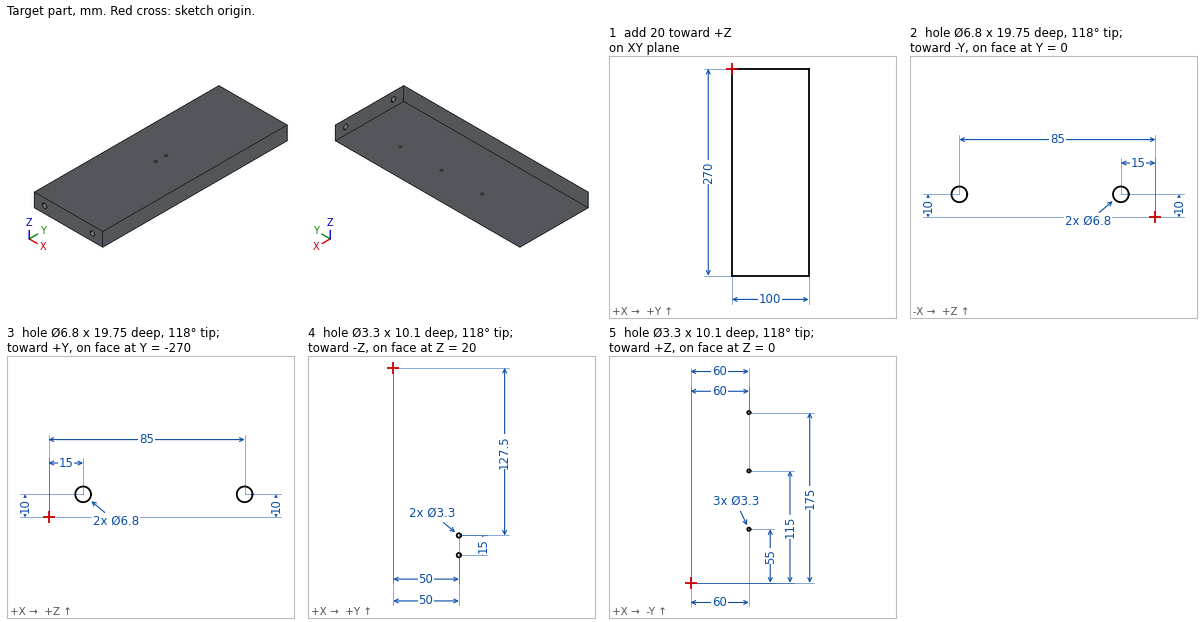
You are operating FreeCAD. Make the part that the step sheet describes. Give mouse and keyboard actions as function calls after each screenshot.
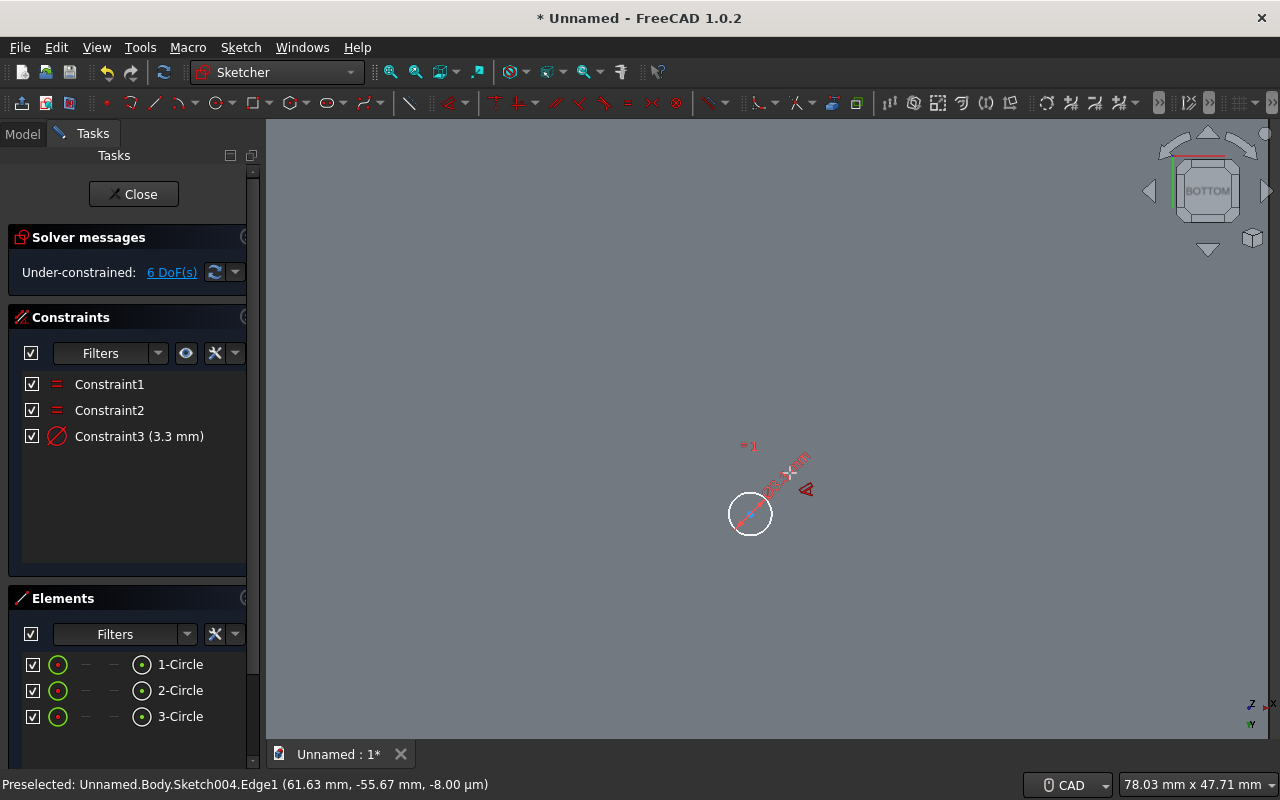
scroll(771, 499, down, 9)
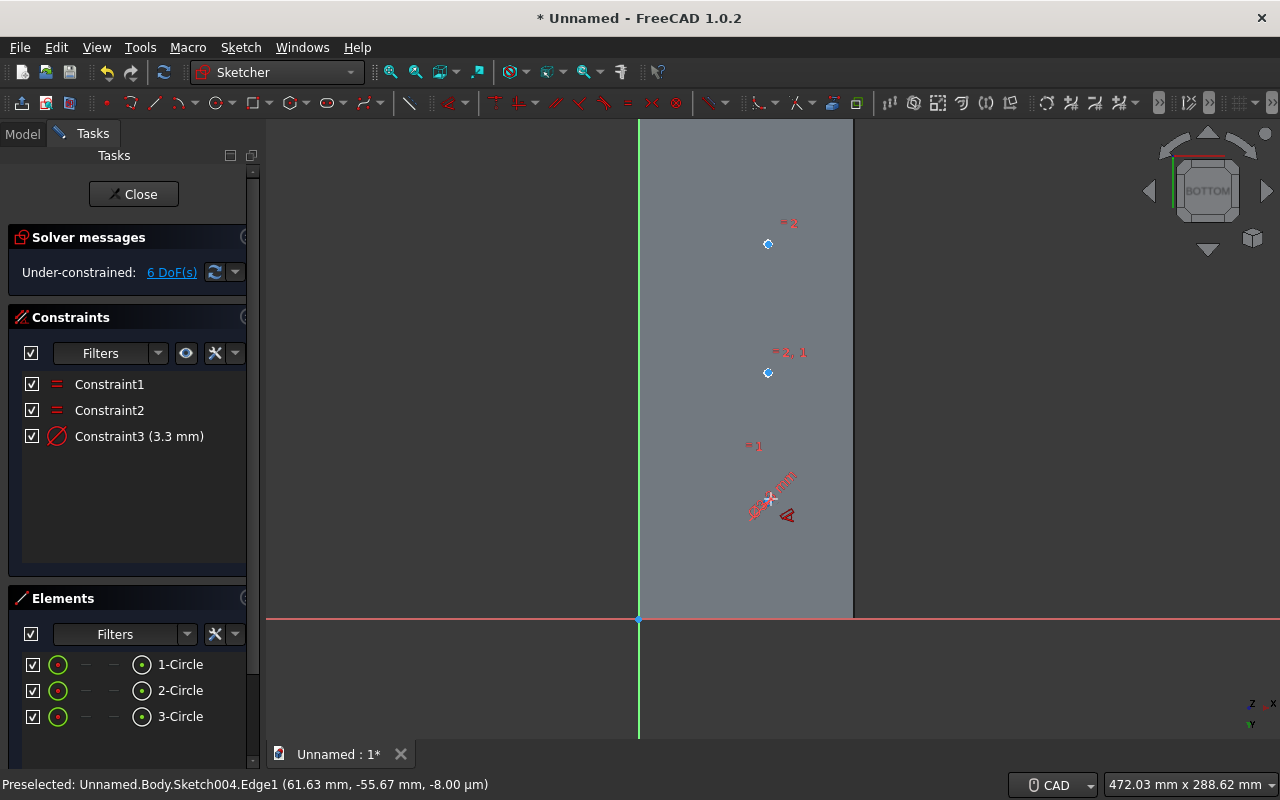
click(768, 502)
click(703, 653)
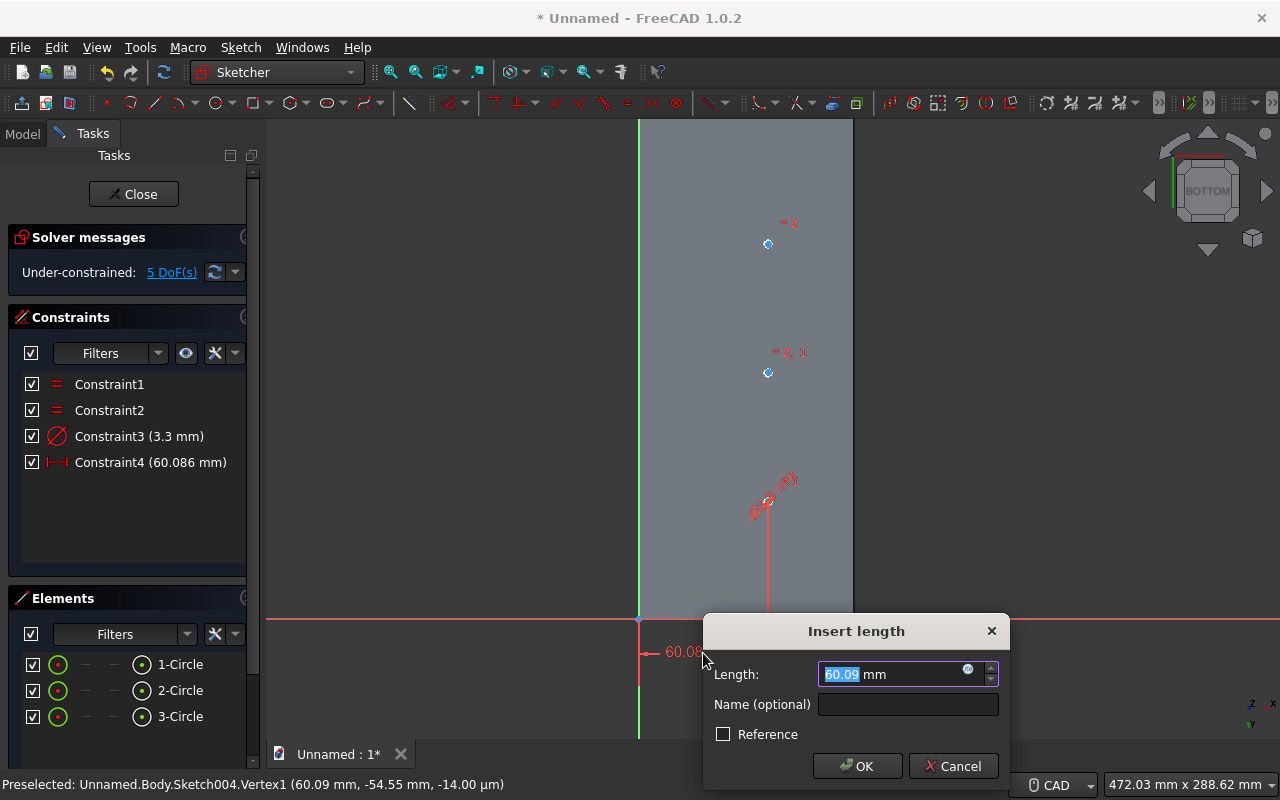
text(60)
key(Return)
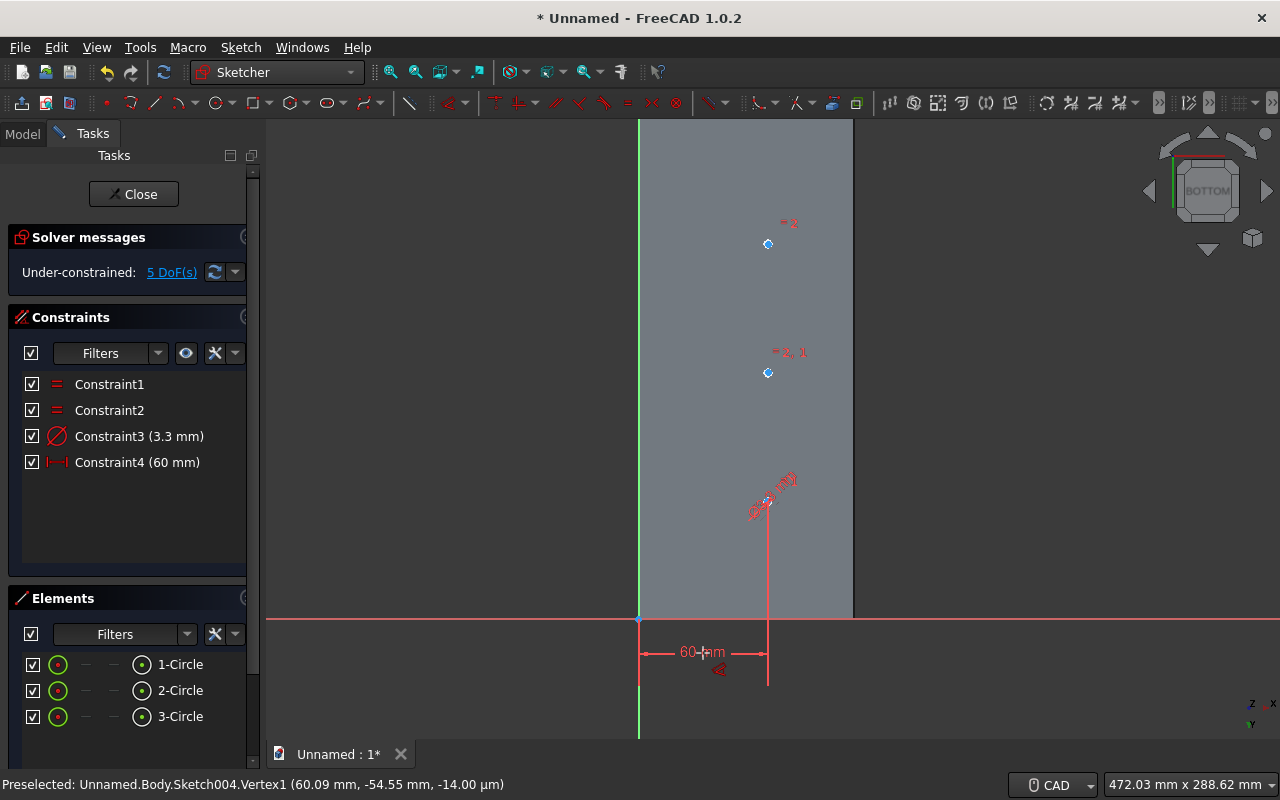
click(768, 502)
click(605, 561)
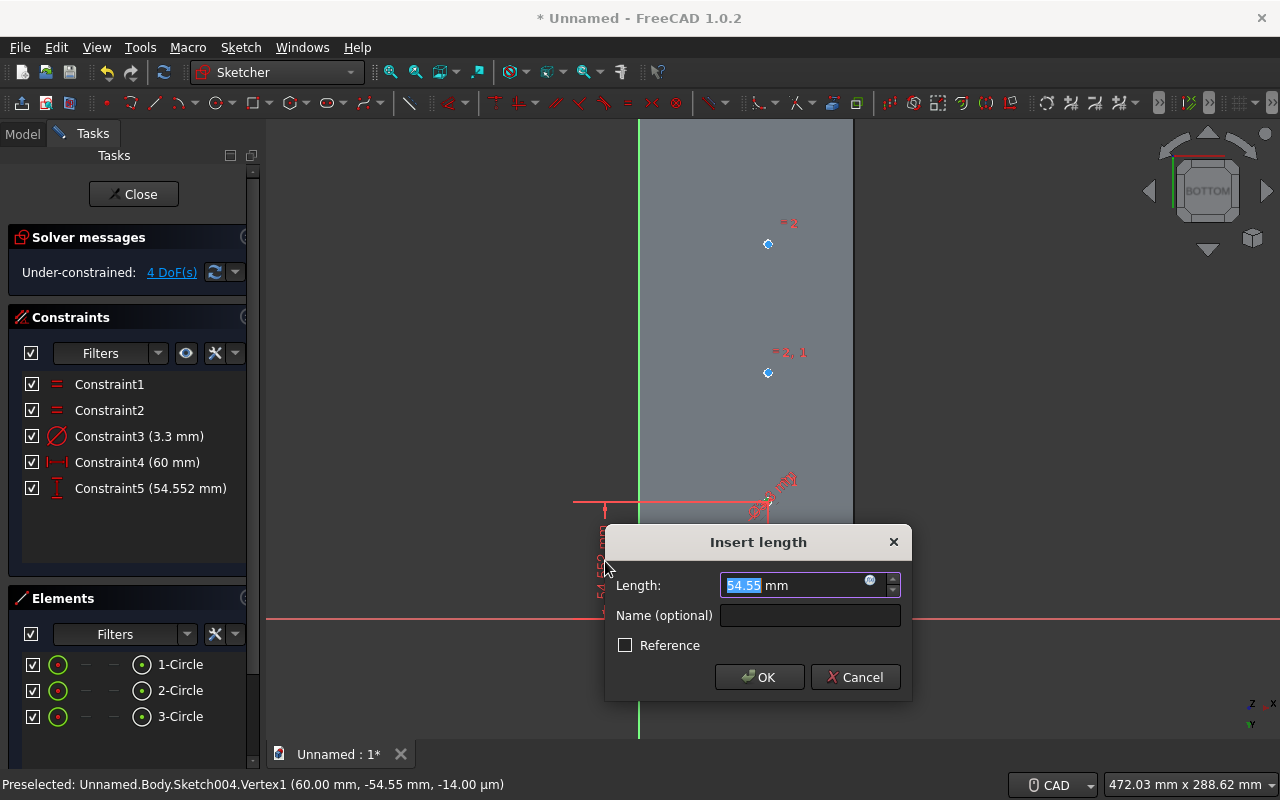
text(55)
key(Return)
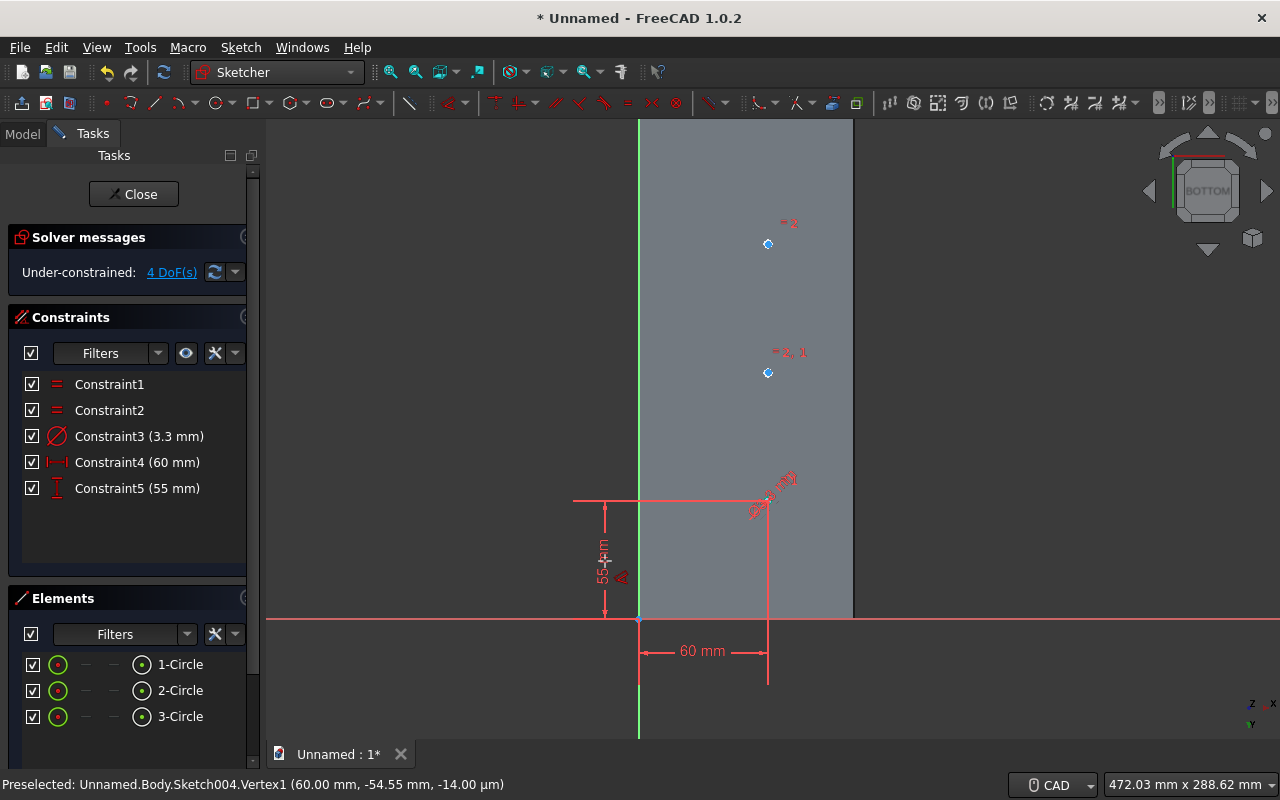
click(768, 373)
click(703, 339)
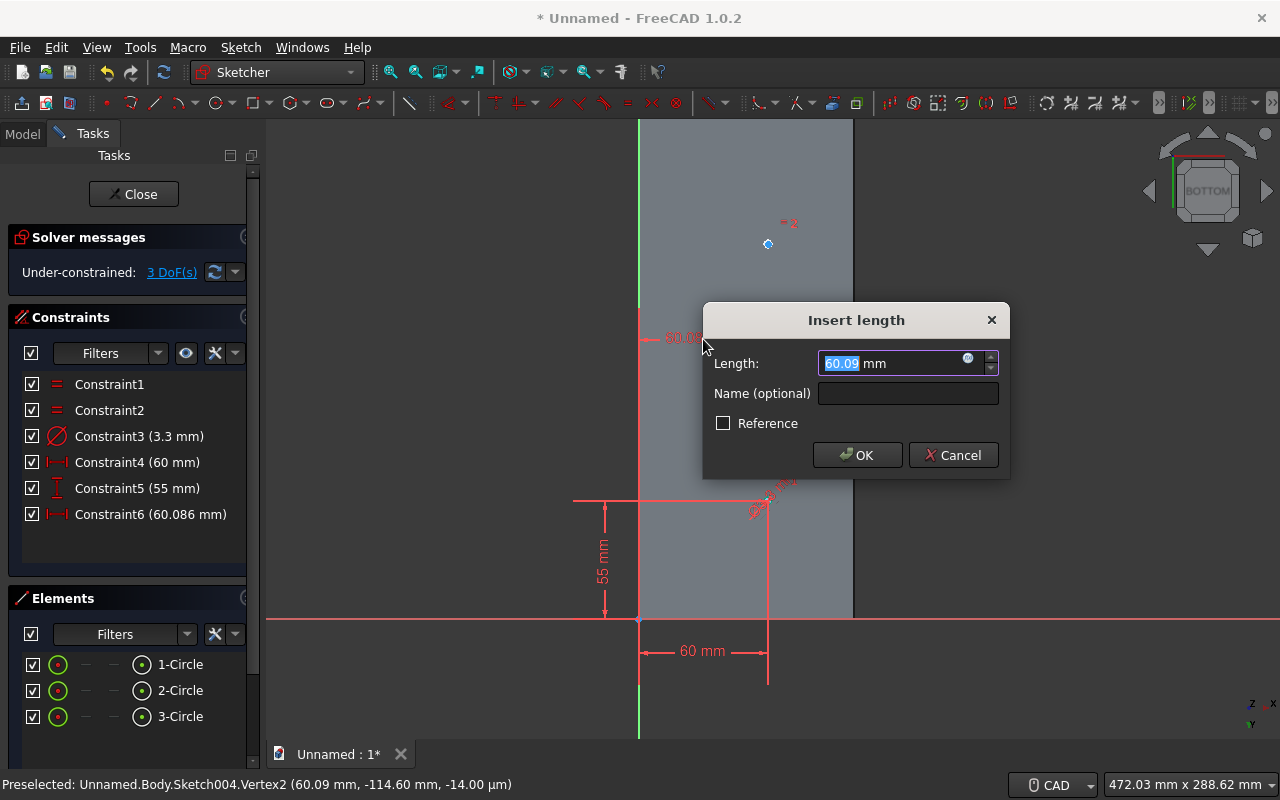
text(60)
key(Return)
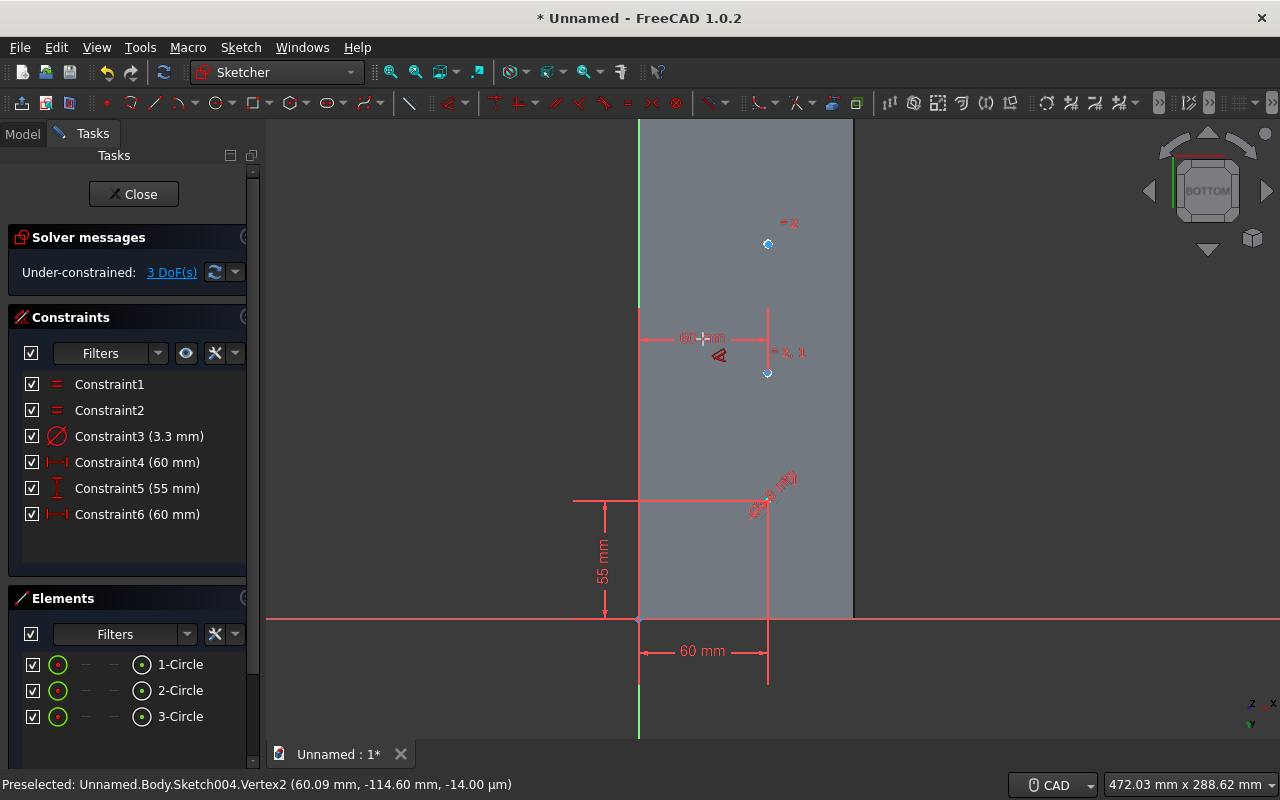
click(768, 244)
click(703, 210)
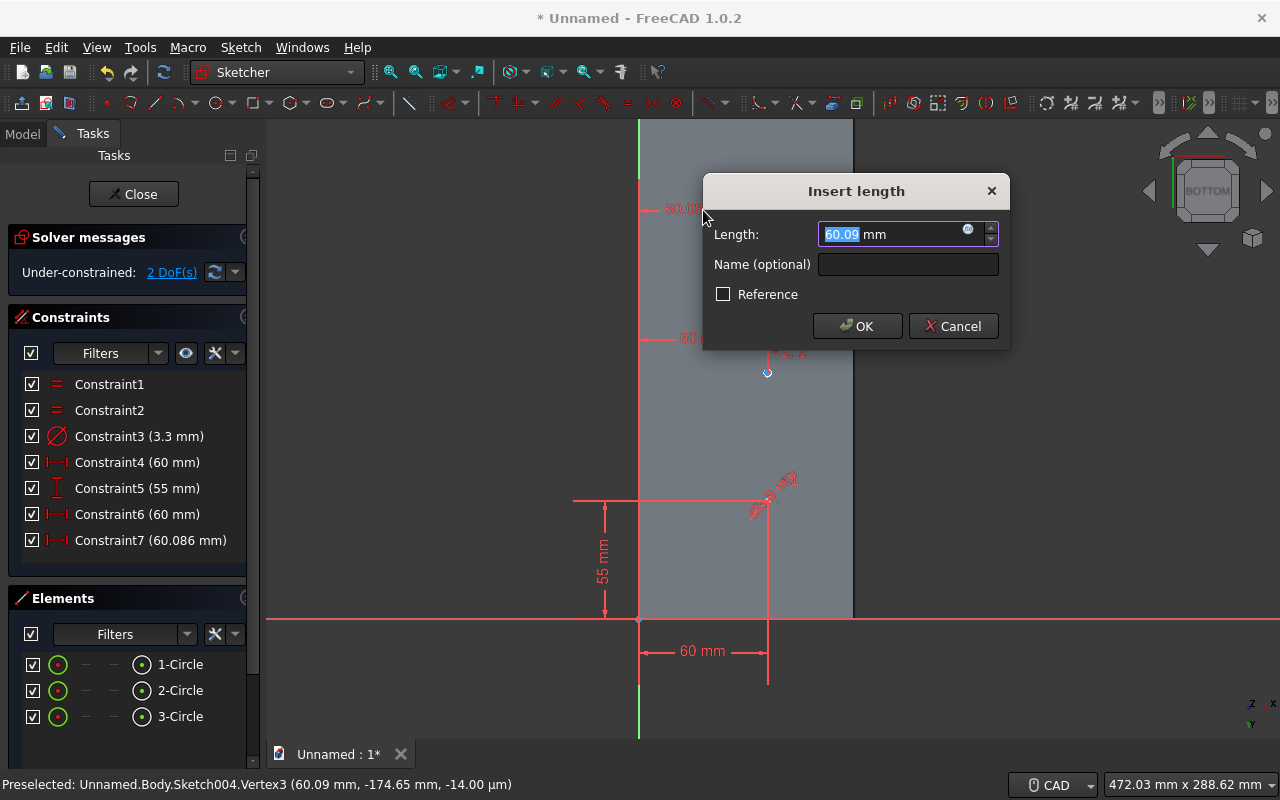
text(60)
key(Return)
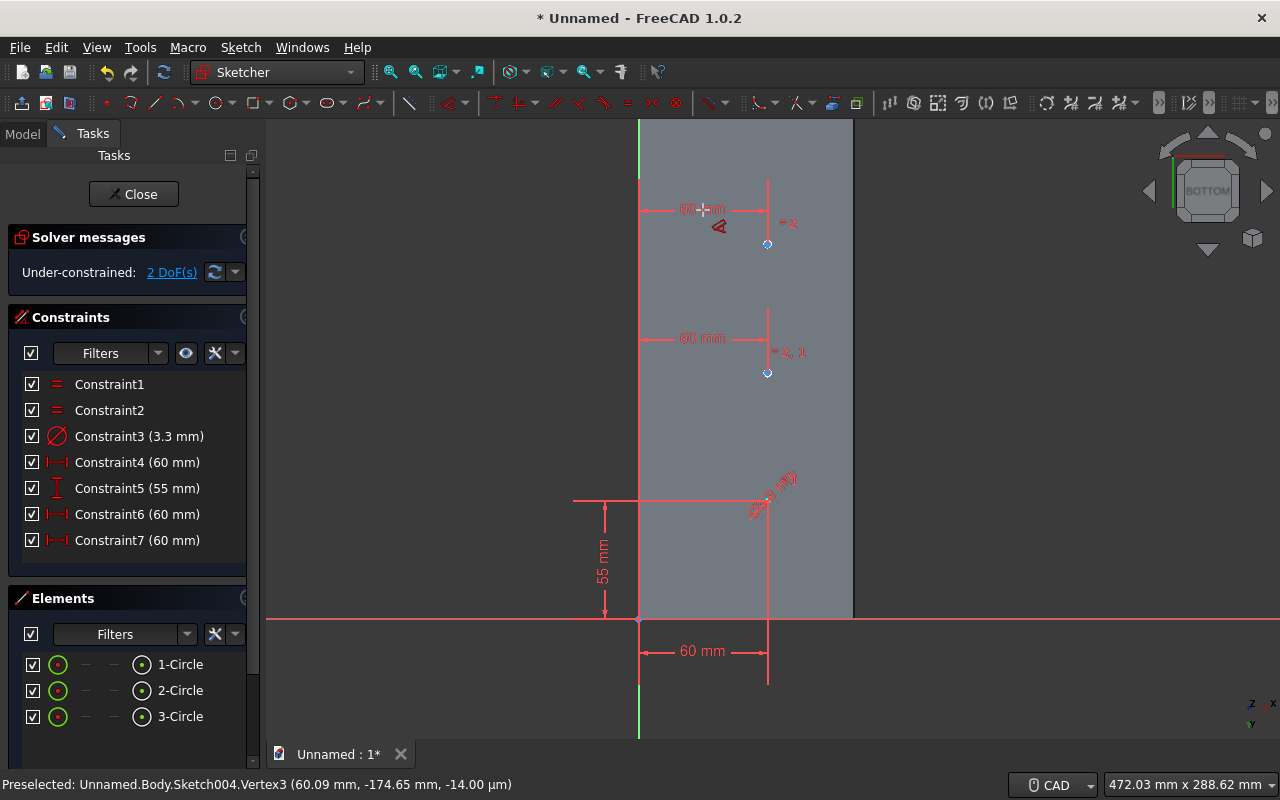
click(768, 373)
click(605, 496)